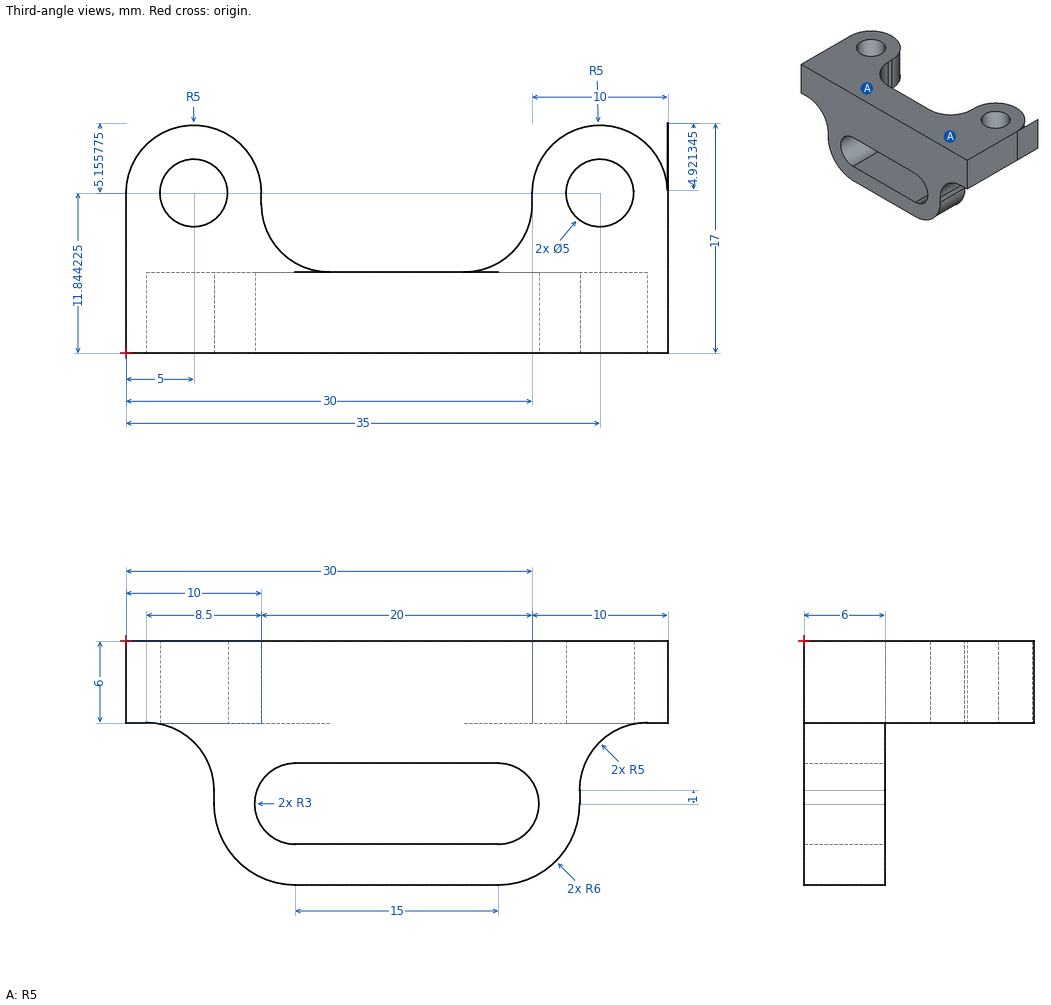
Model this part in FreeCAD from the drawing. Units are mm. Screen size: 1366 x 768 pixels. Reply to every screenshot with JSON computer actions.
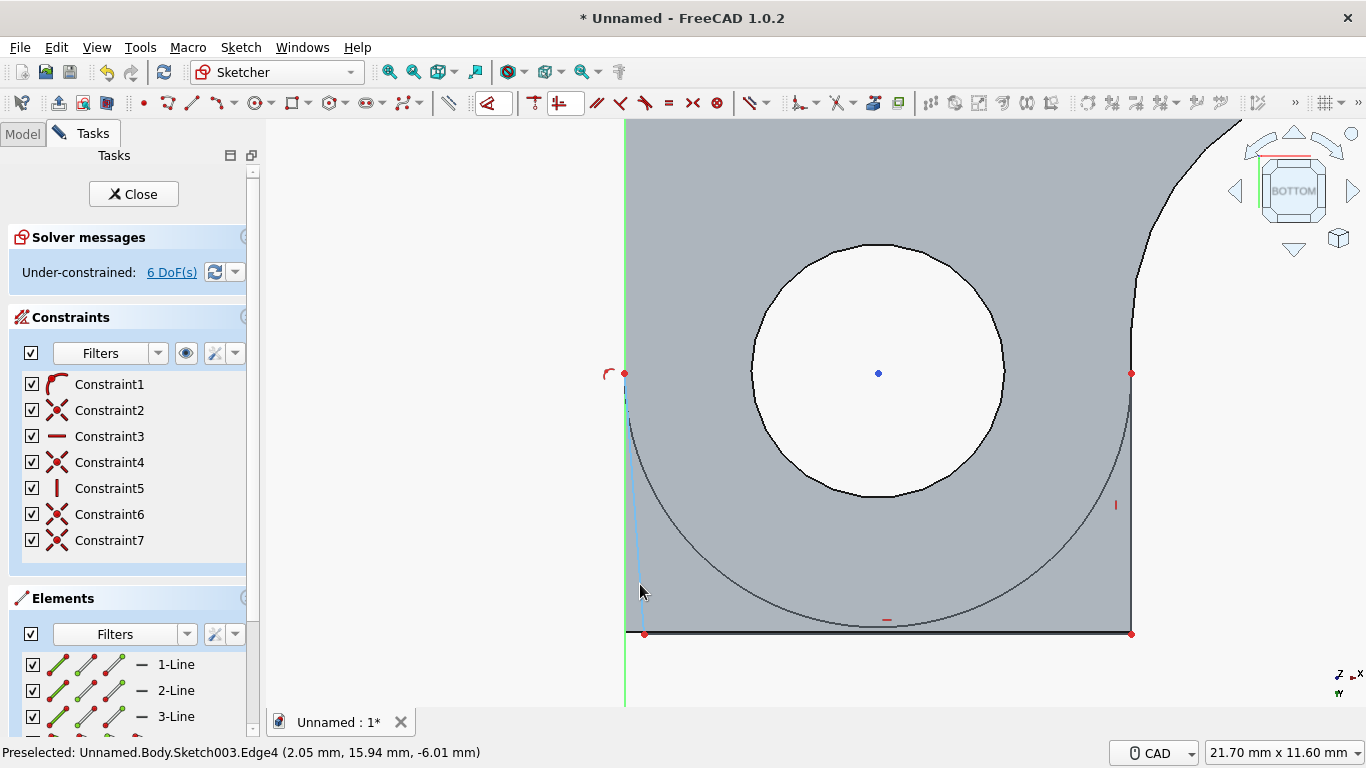
{"action": "left_click", "coordinate": [640, 582]}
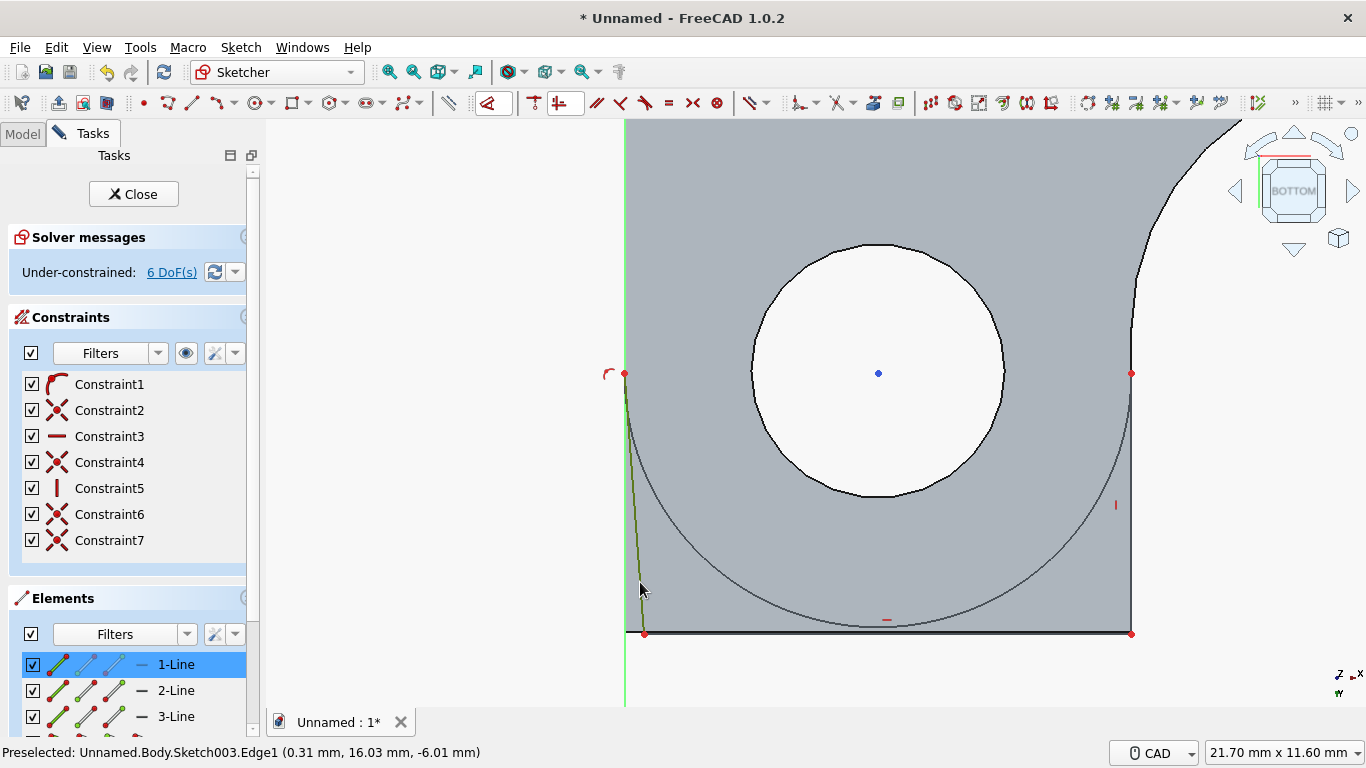
{"action": "left_click", "coordinate": [729, 579]}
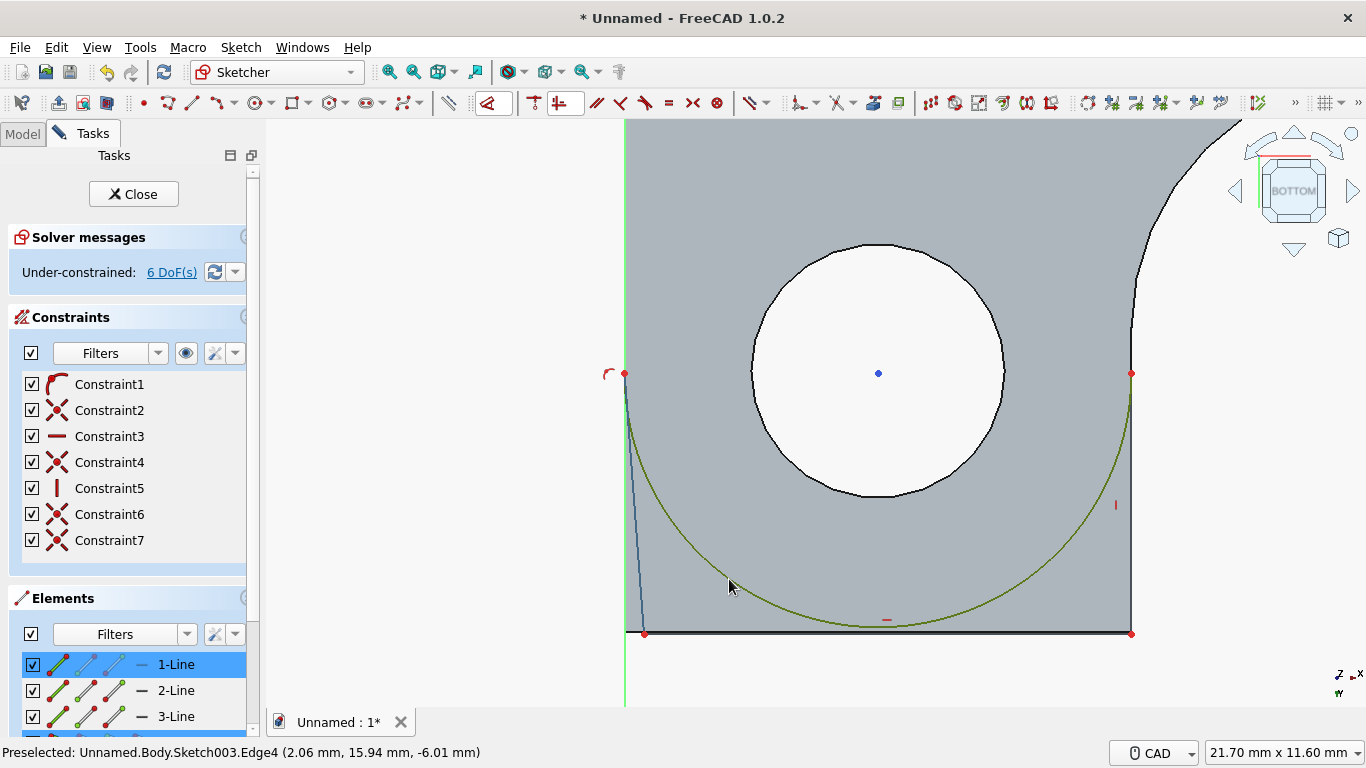
{"action": "key", "text": "t"}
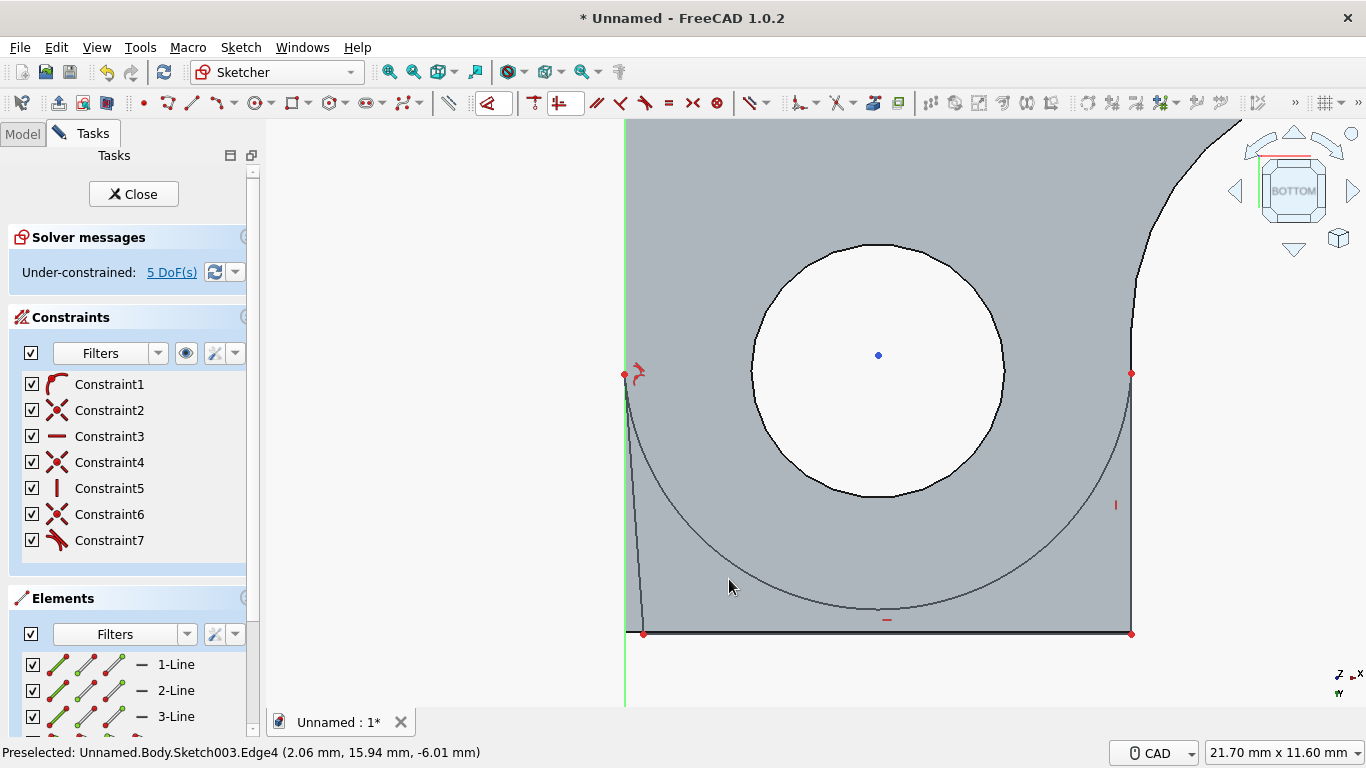
{"action": "left_click", "coordinate": [1131, 556]}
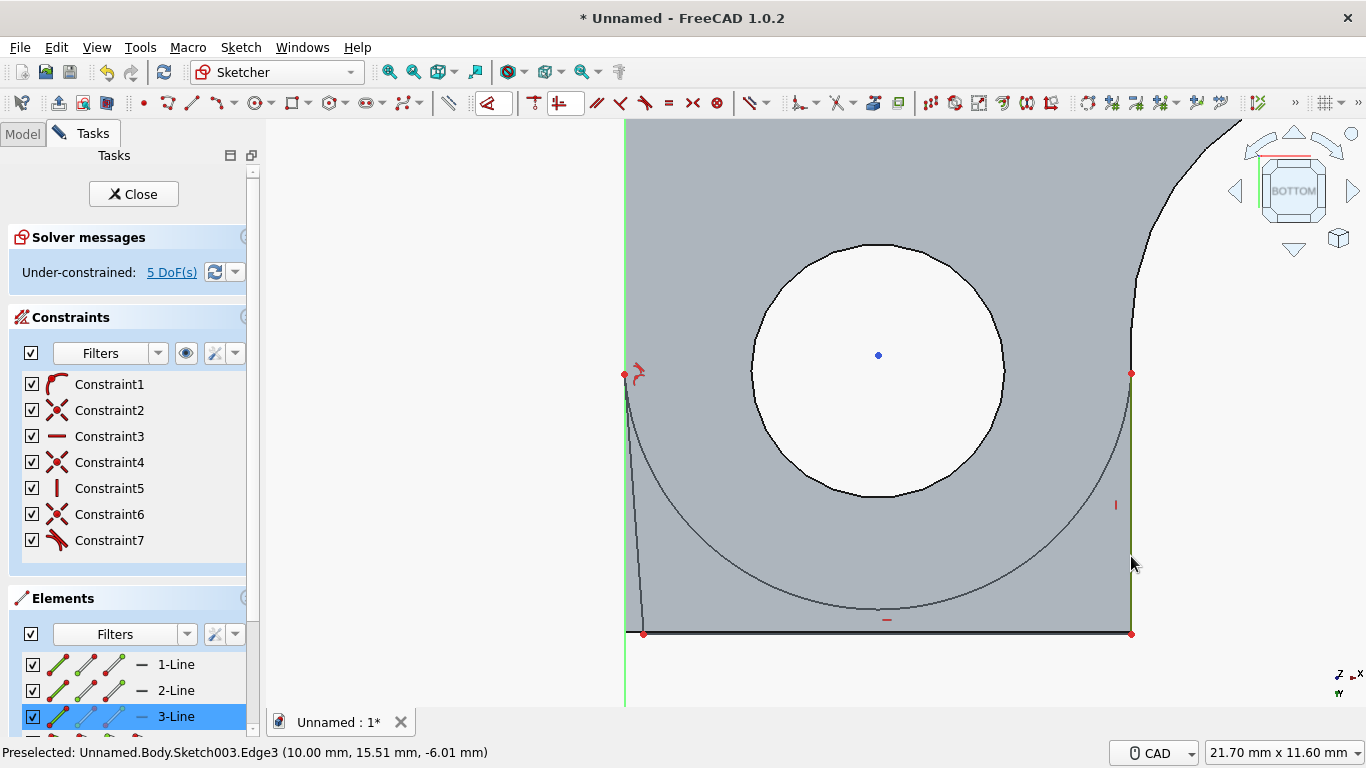
{"action": "left_click", "coordinate": [735, 565]}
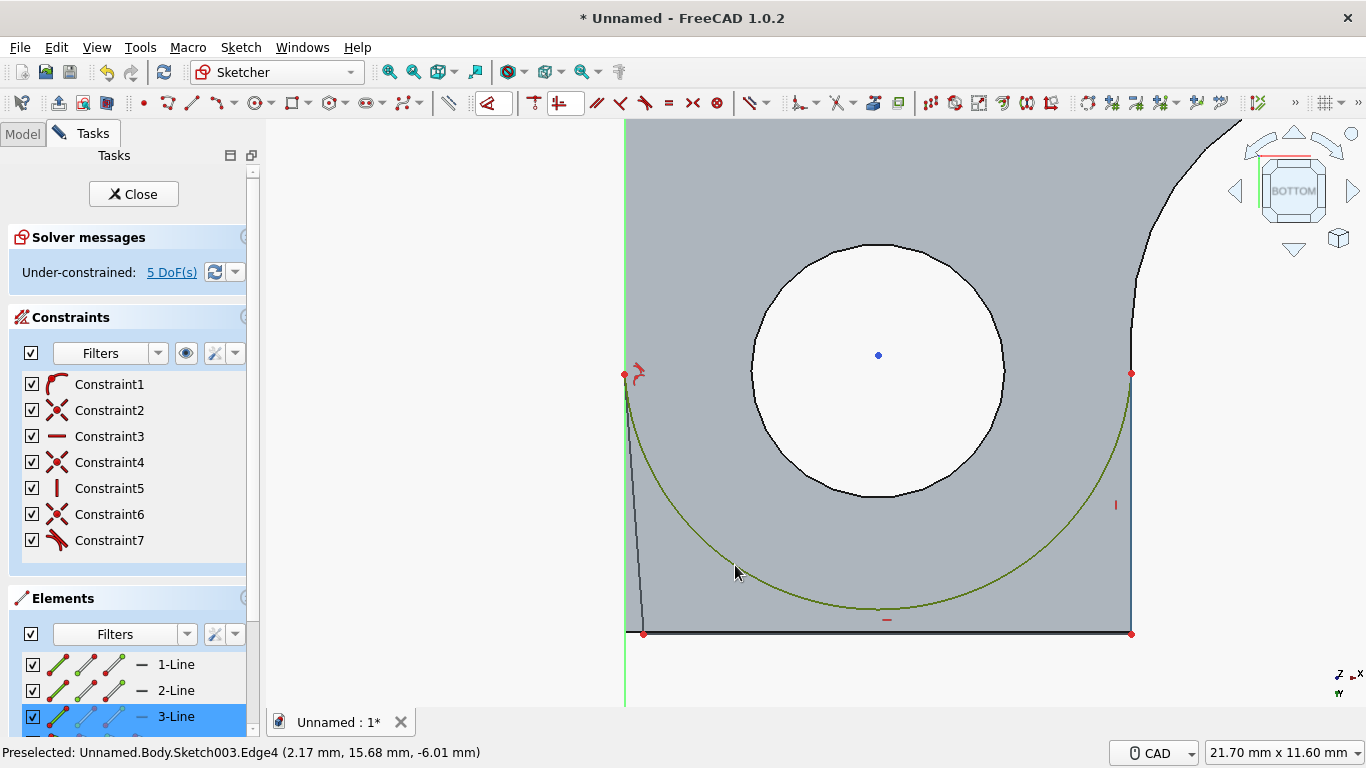
{"action": "key", "text": "t"}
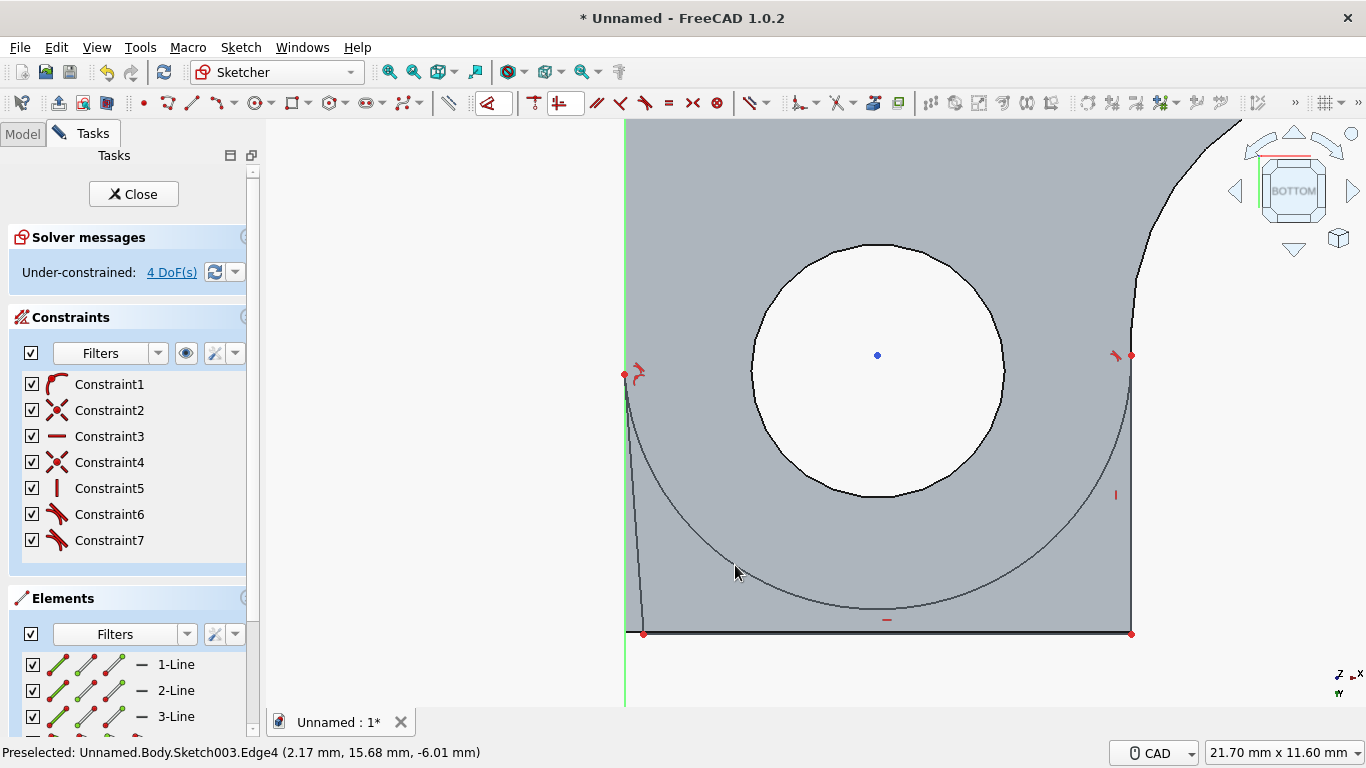
{"action": "left_click", "coordinate": [638, 556]}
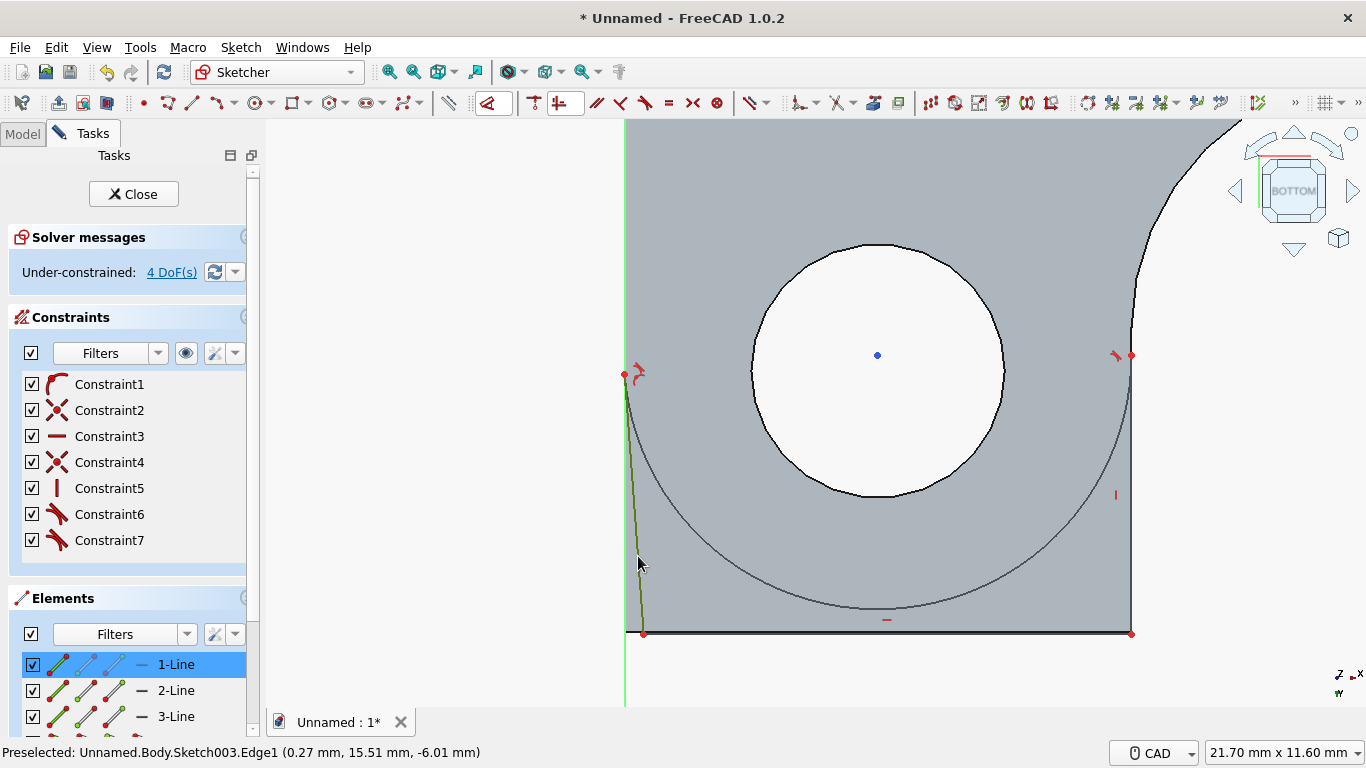
{"action": "key", "text": "v"}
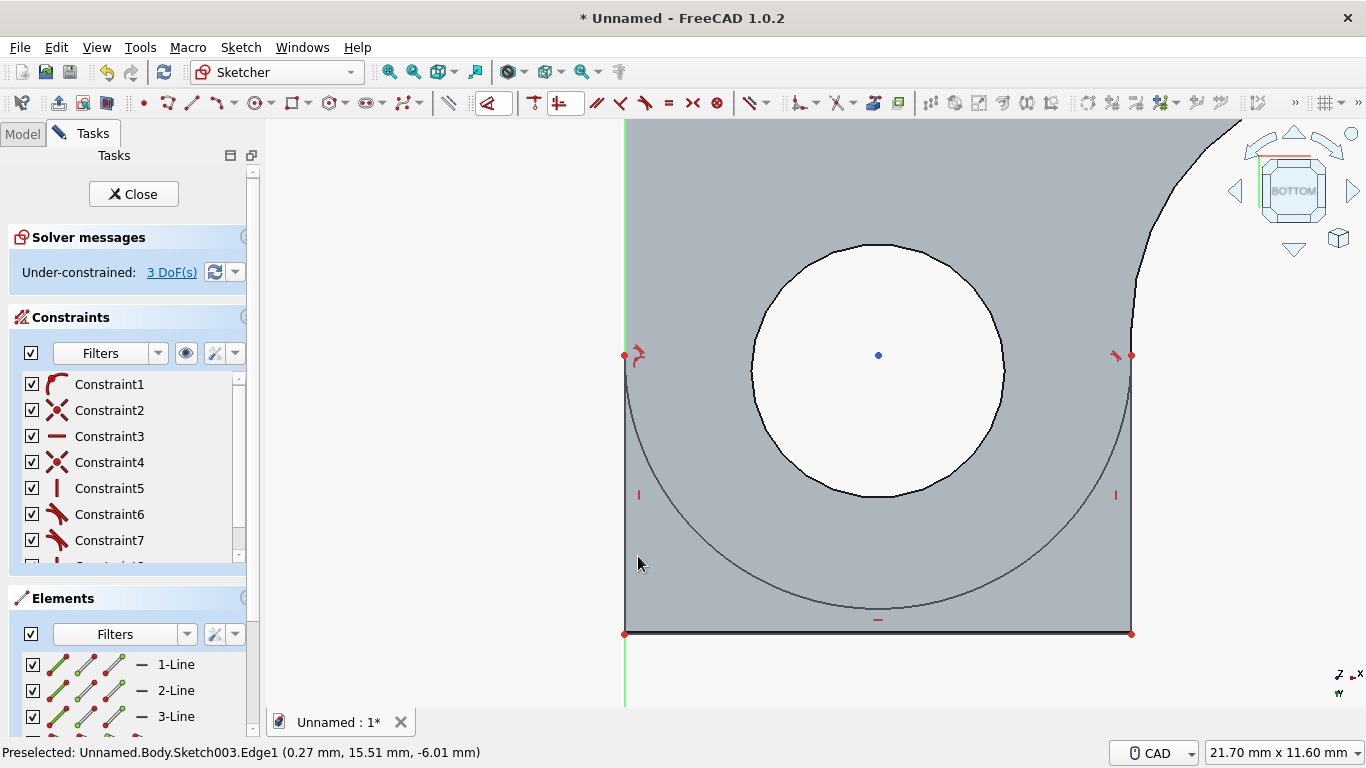
{"action": "left_click", "coordinate": [729, 561]}